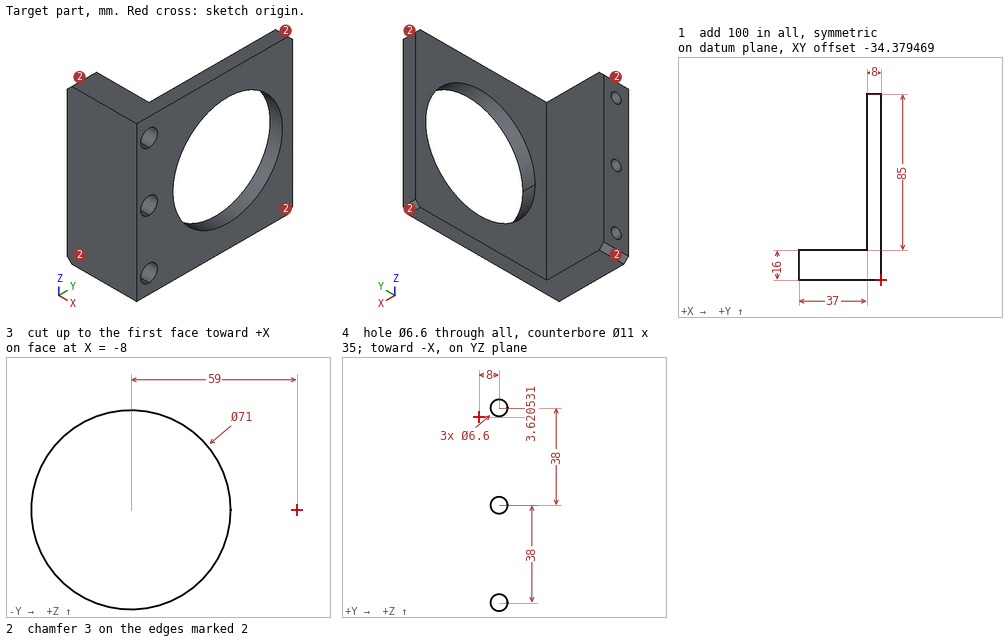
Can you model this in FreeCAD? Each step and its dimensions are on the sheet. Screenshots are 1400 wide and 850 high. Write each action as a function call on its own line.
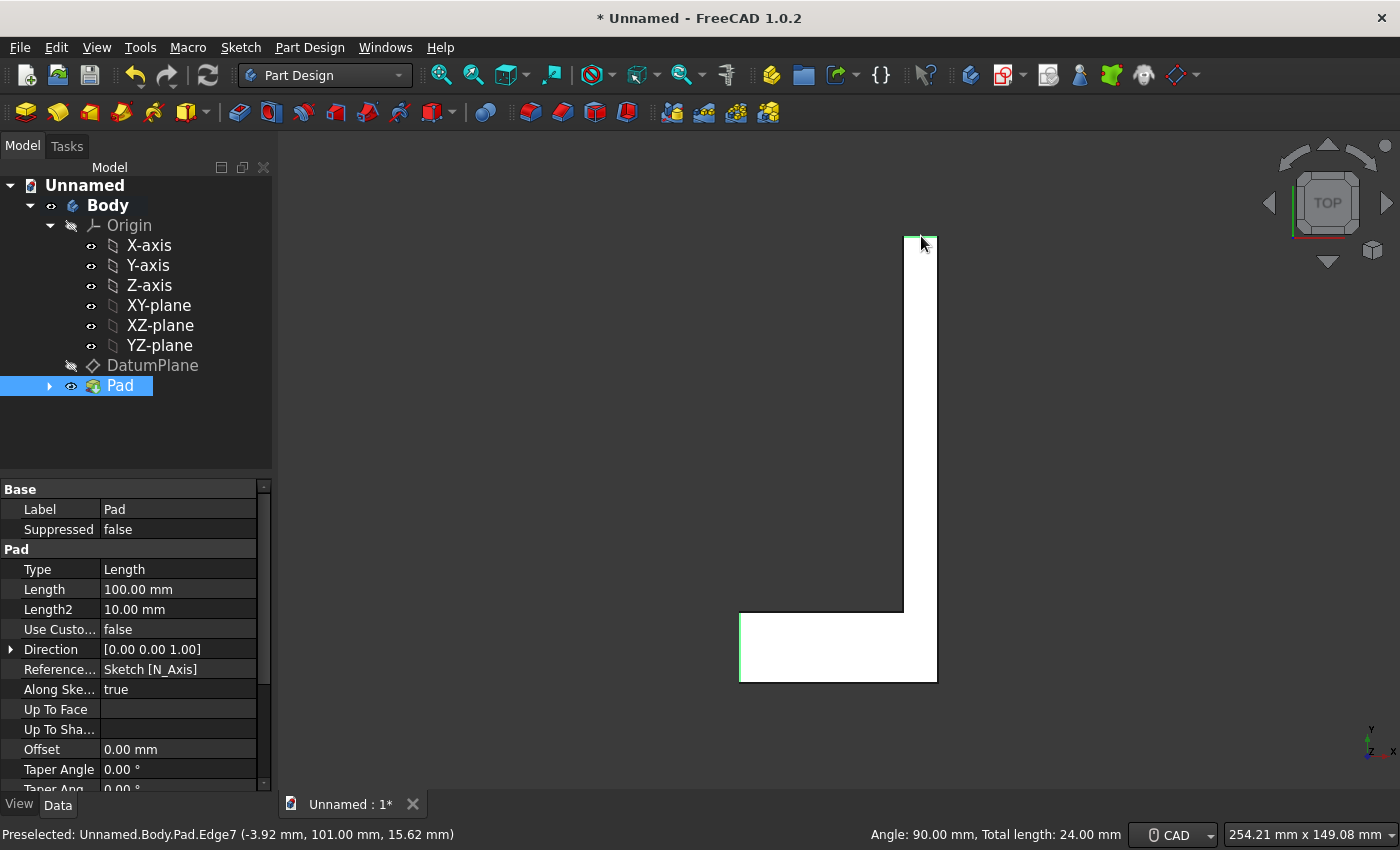
key(1)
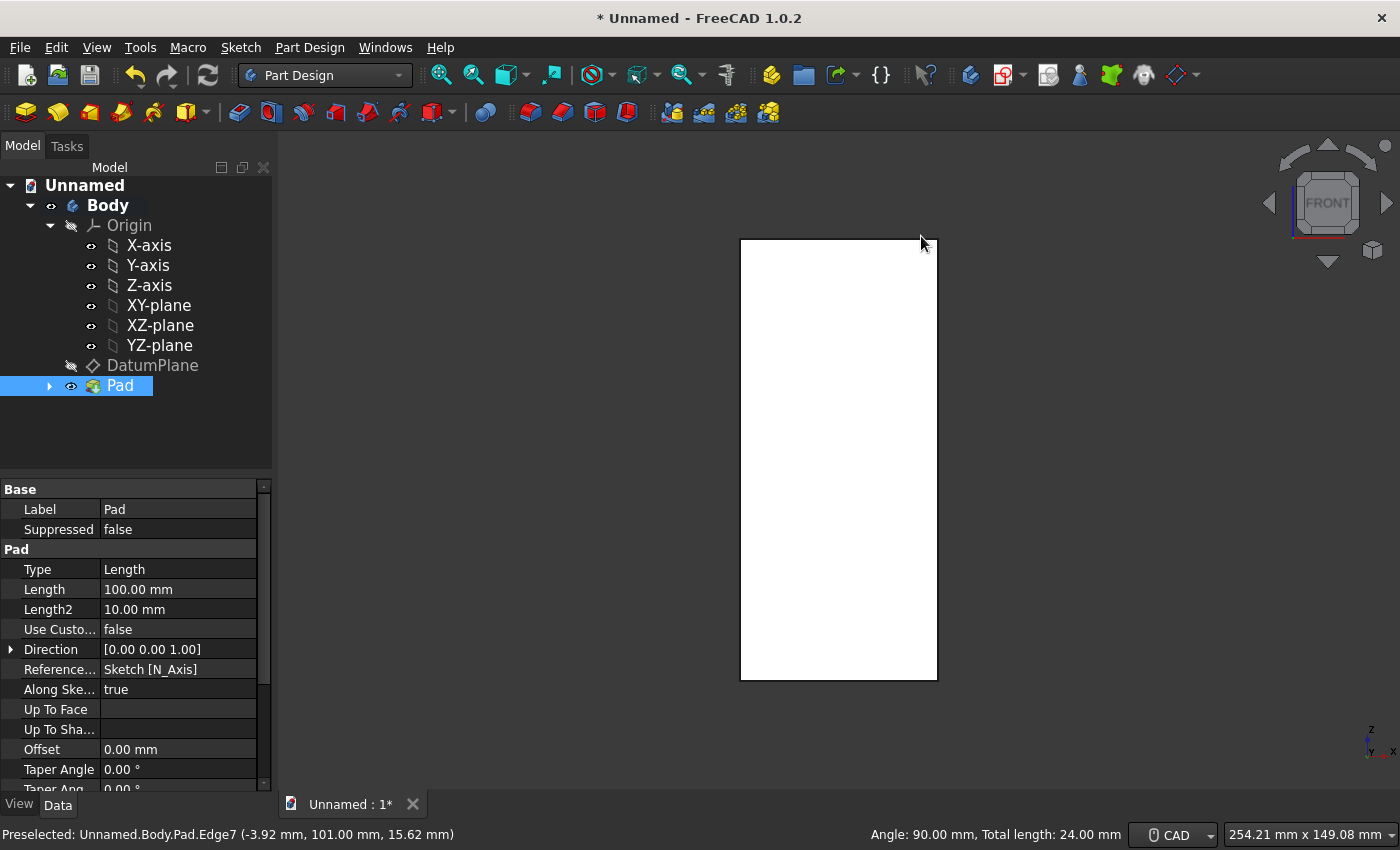
key(3)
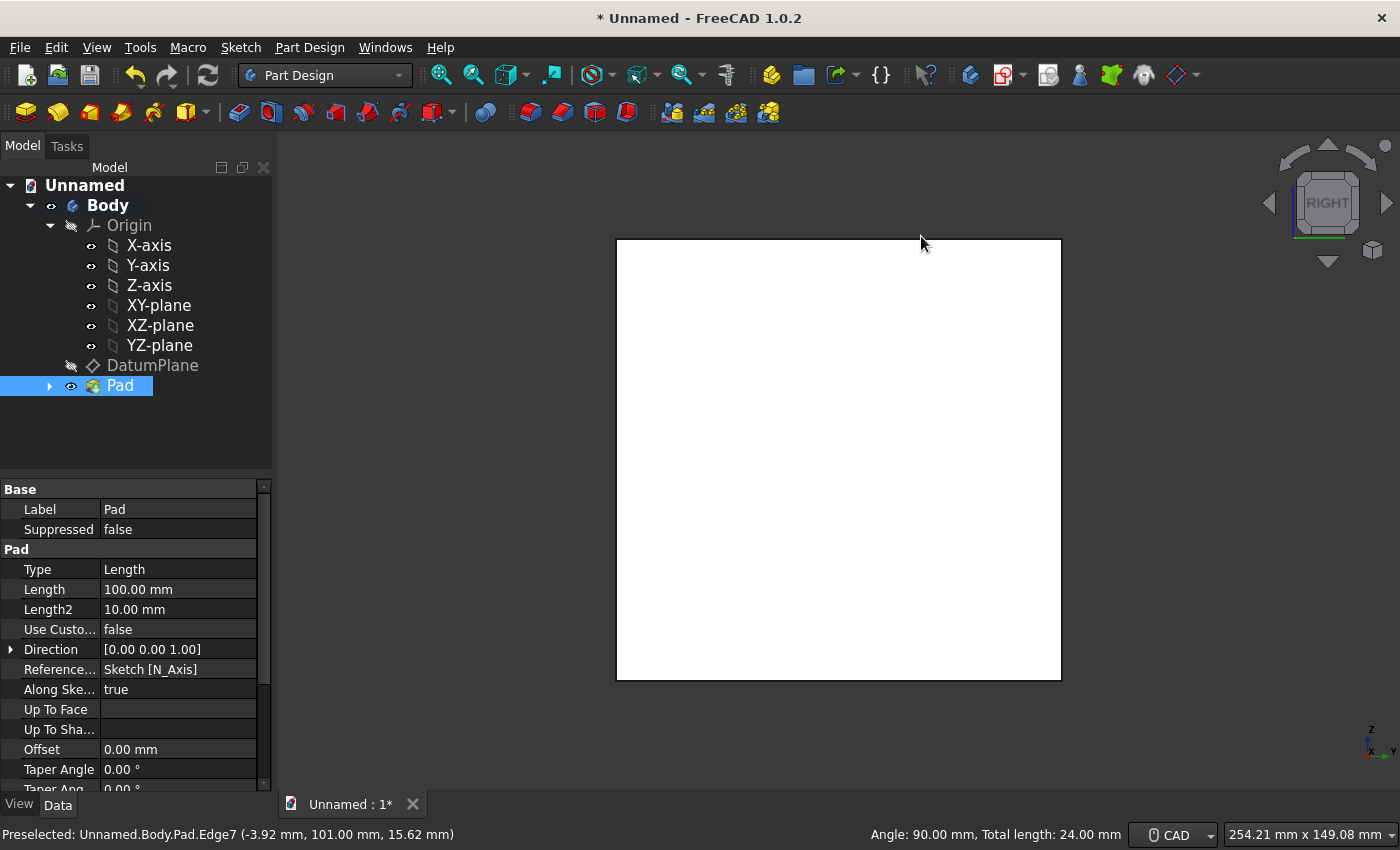
key(5)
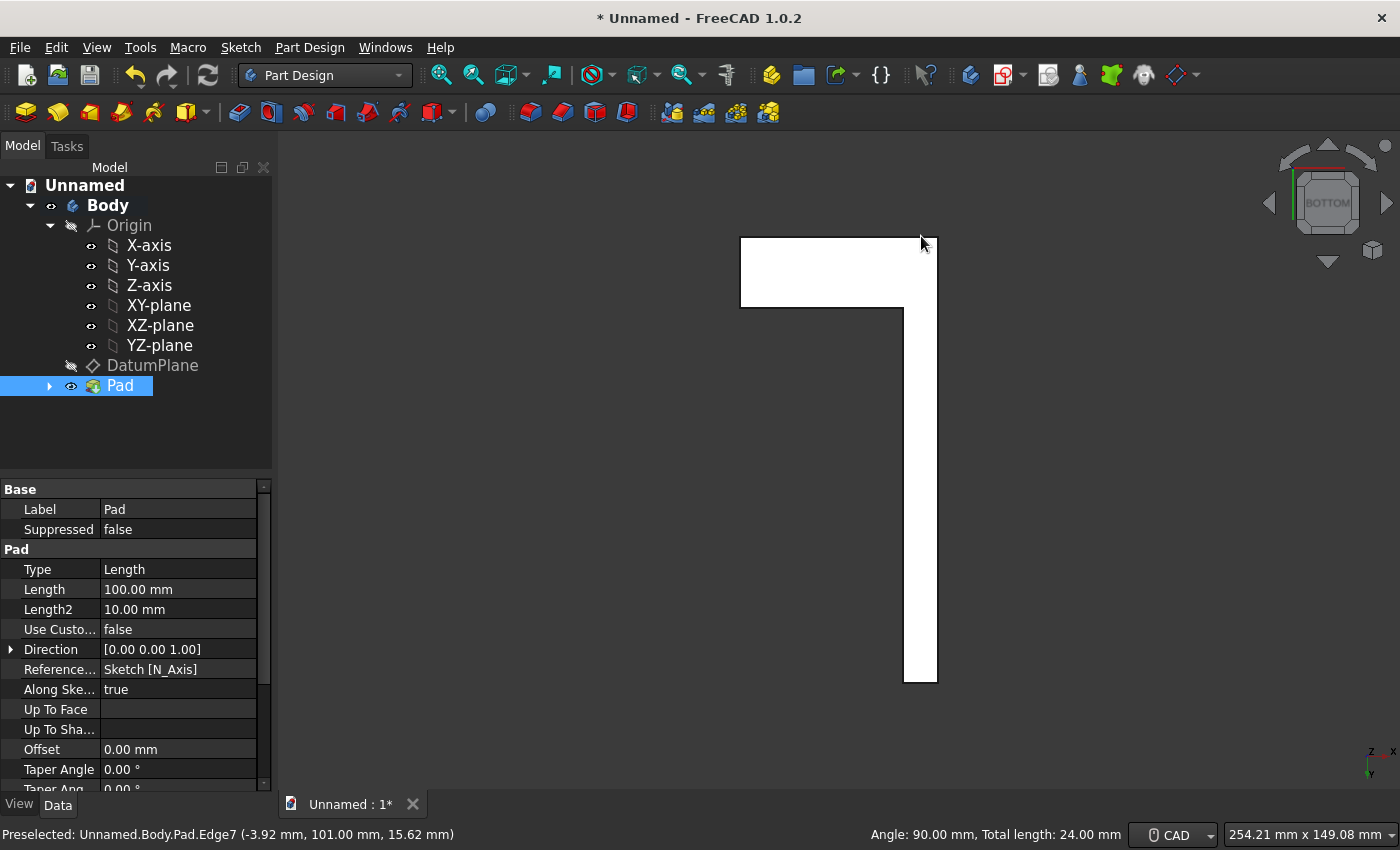
click(740, 271, ctrl)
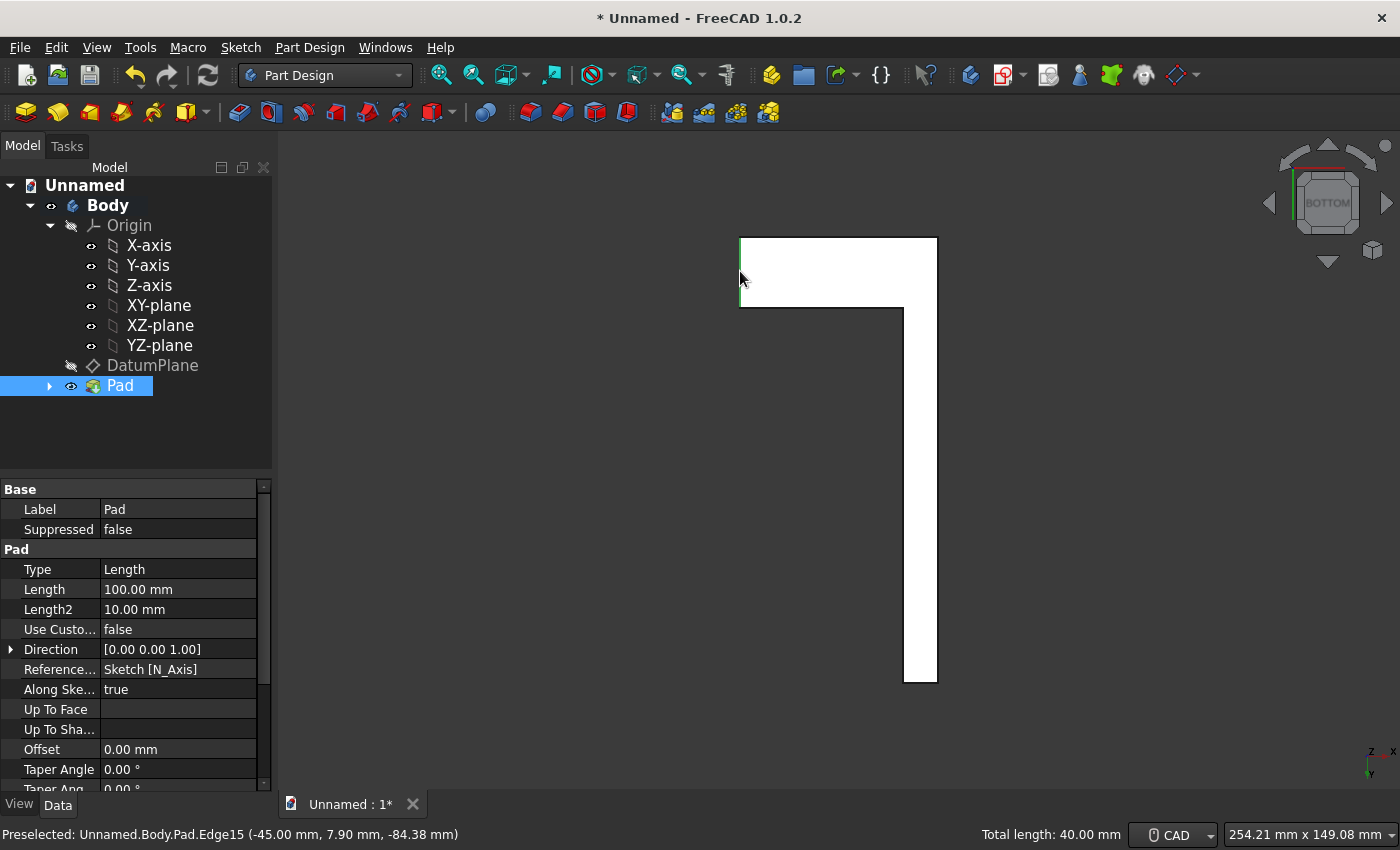
click(921, 682, ctrl)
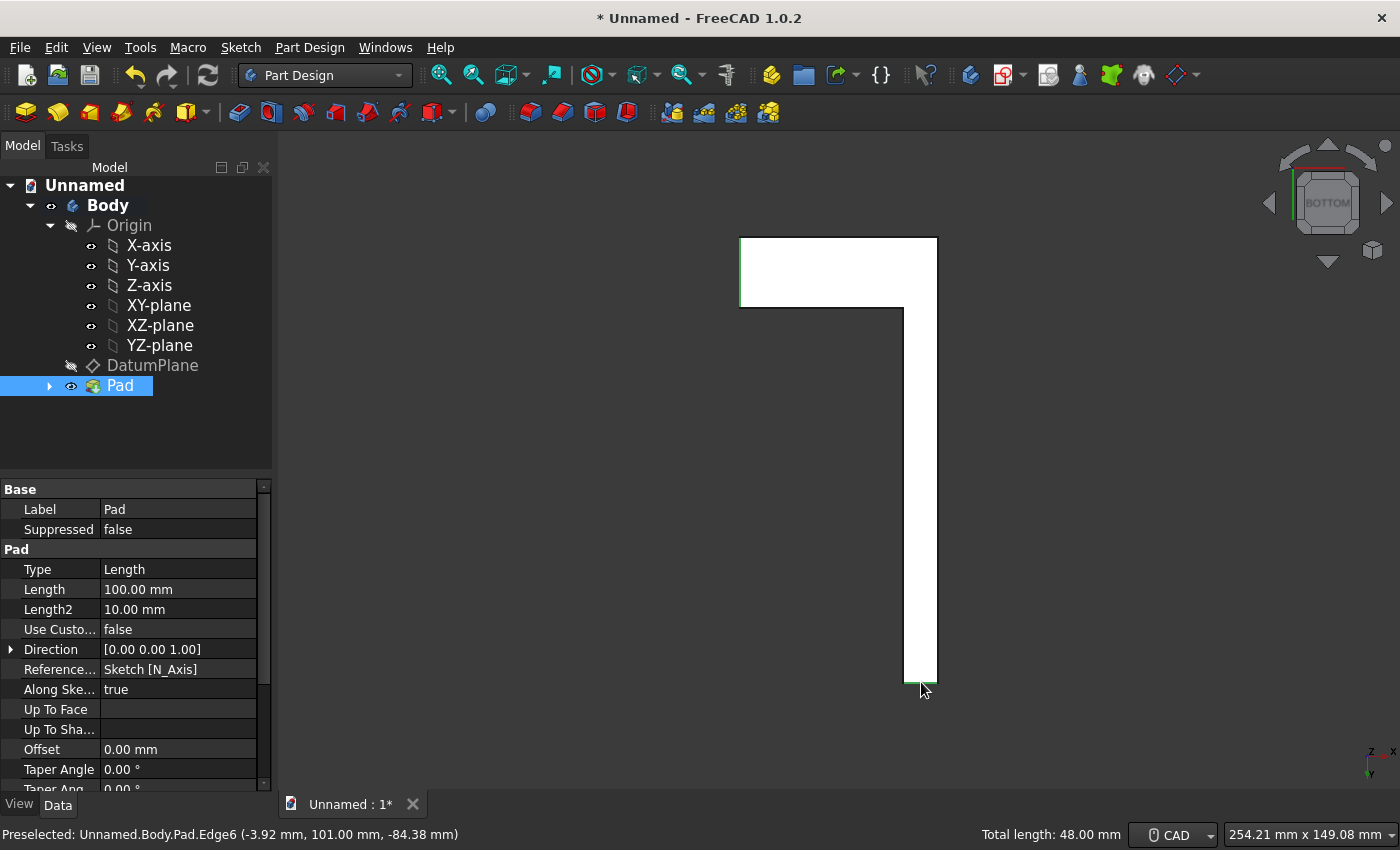
click(564, 112)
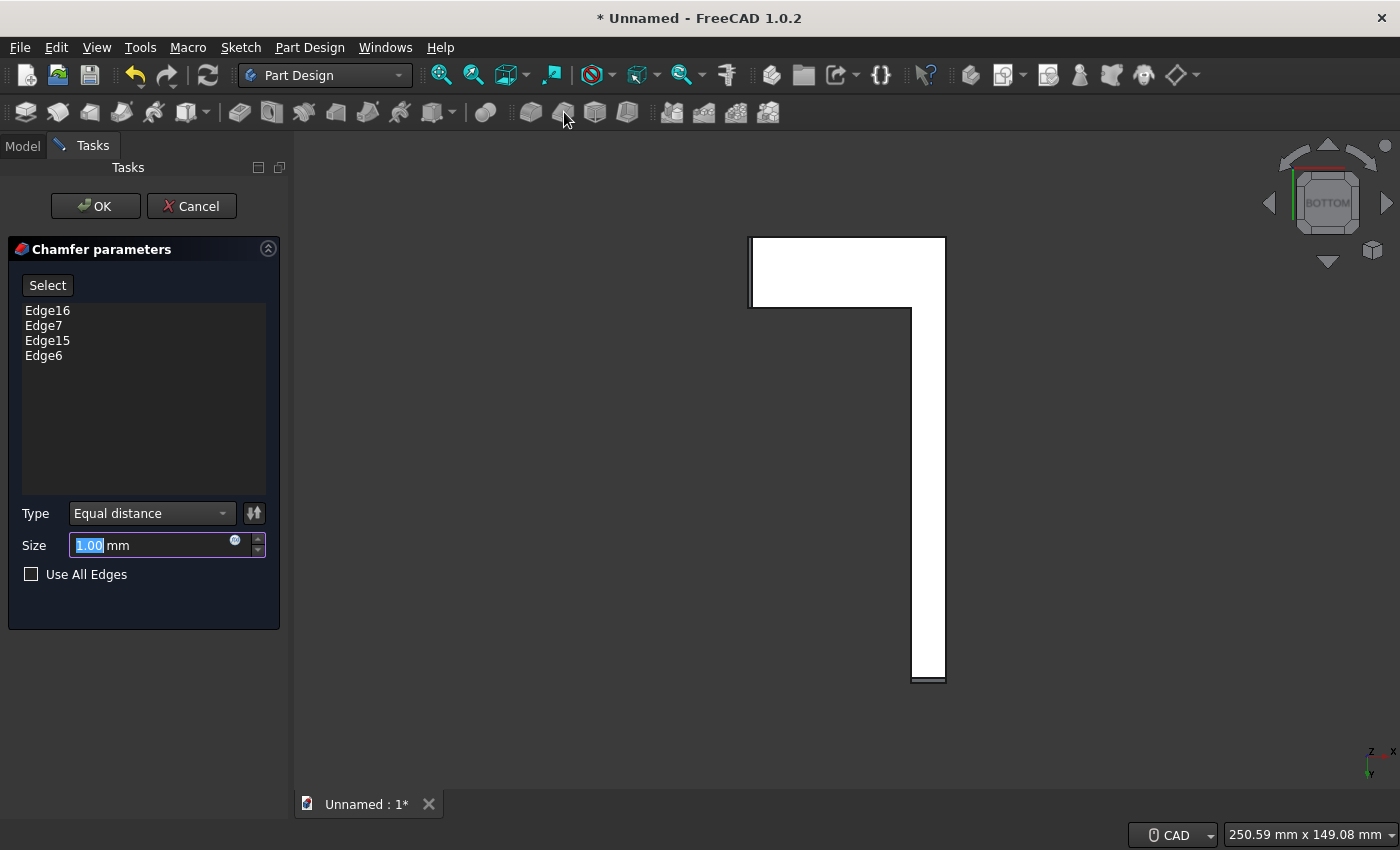
text(3)
key(Tab)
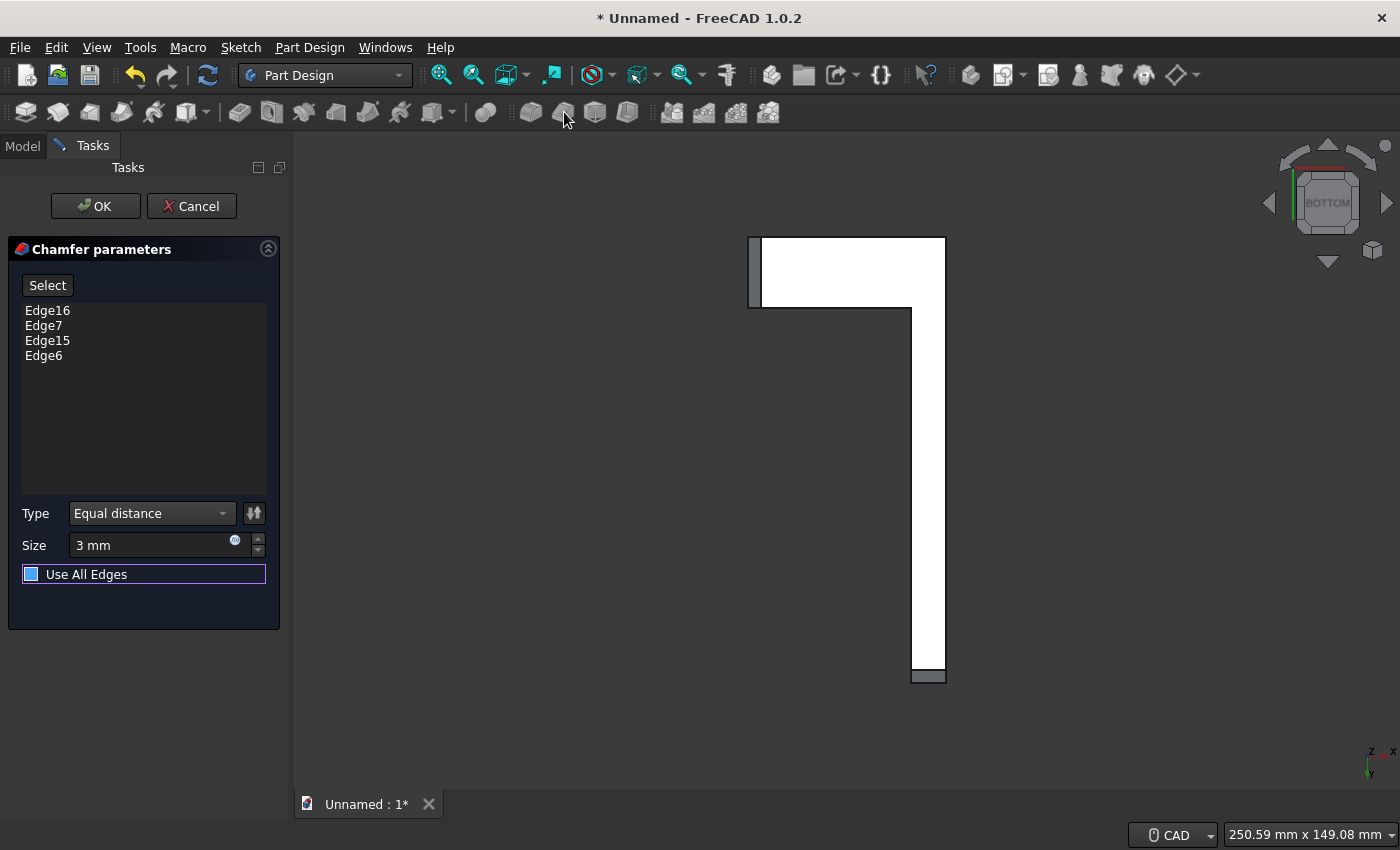
click(96, 206)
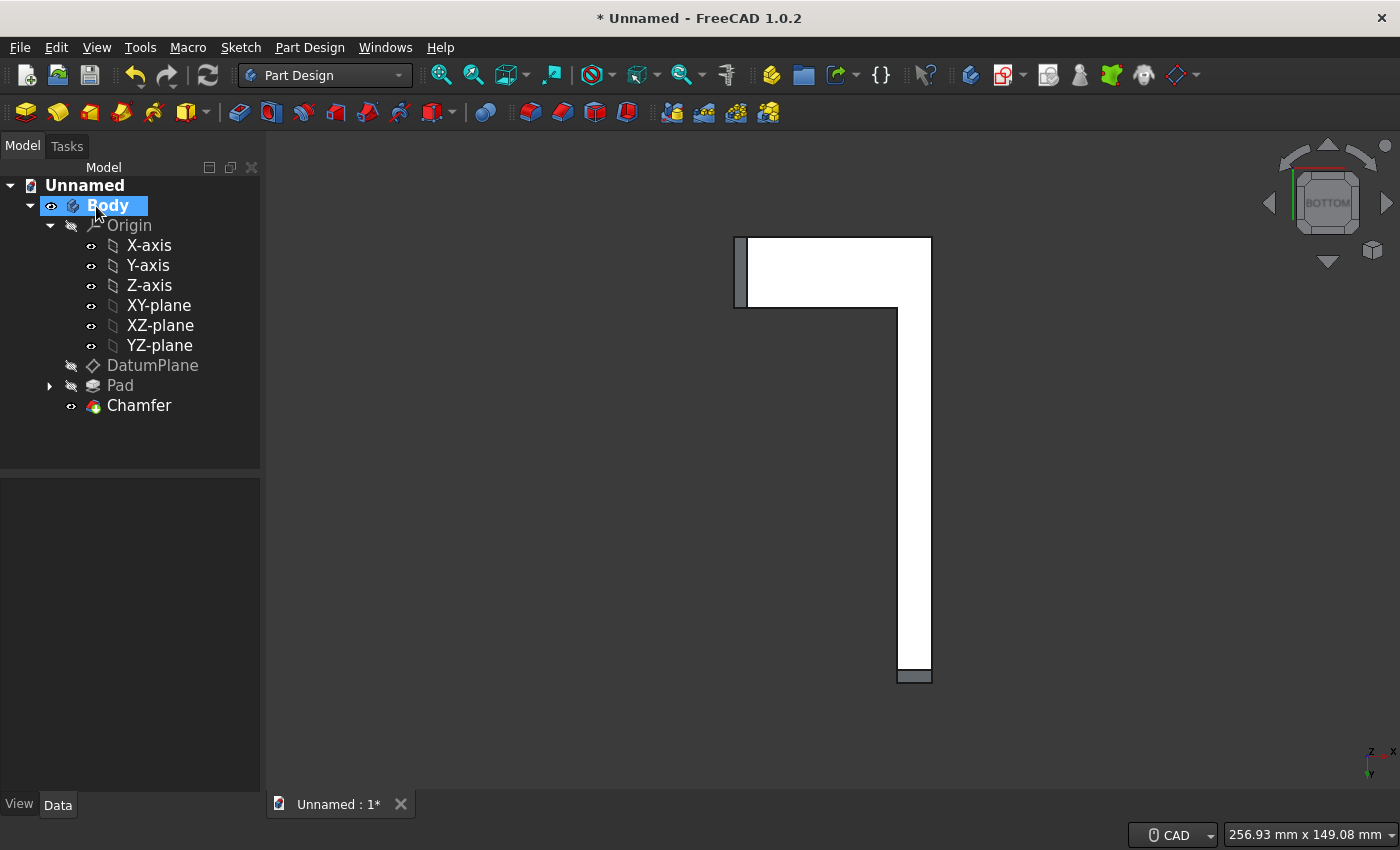
key(6)